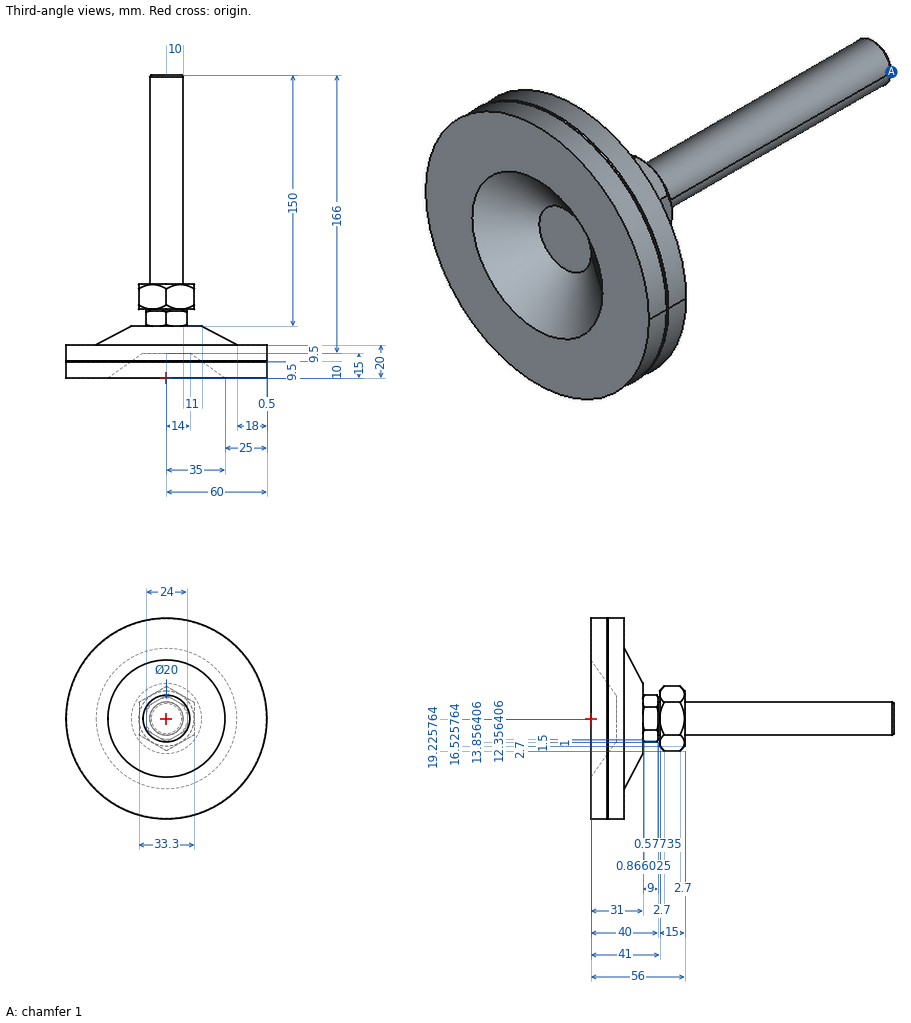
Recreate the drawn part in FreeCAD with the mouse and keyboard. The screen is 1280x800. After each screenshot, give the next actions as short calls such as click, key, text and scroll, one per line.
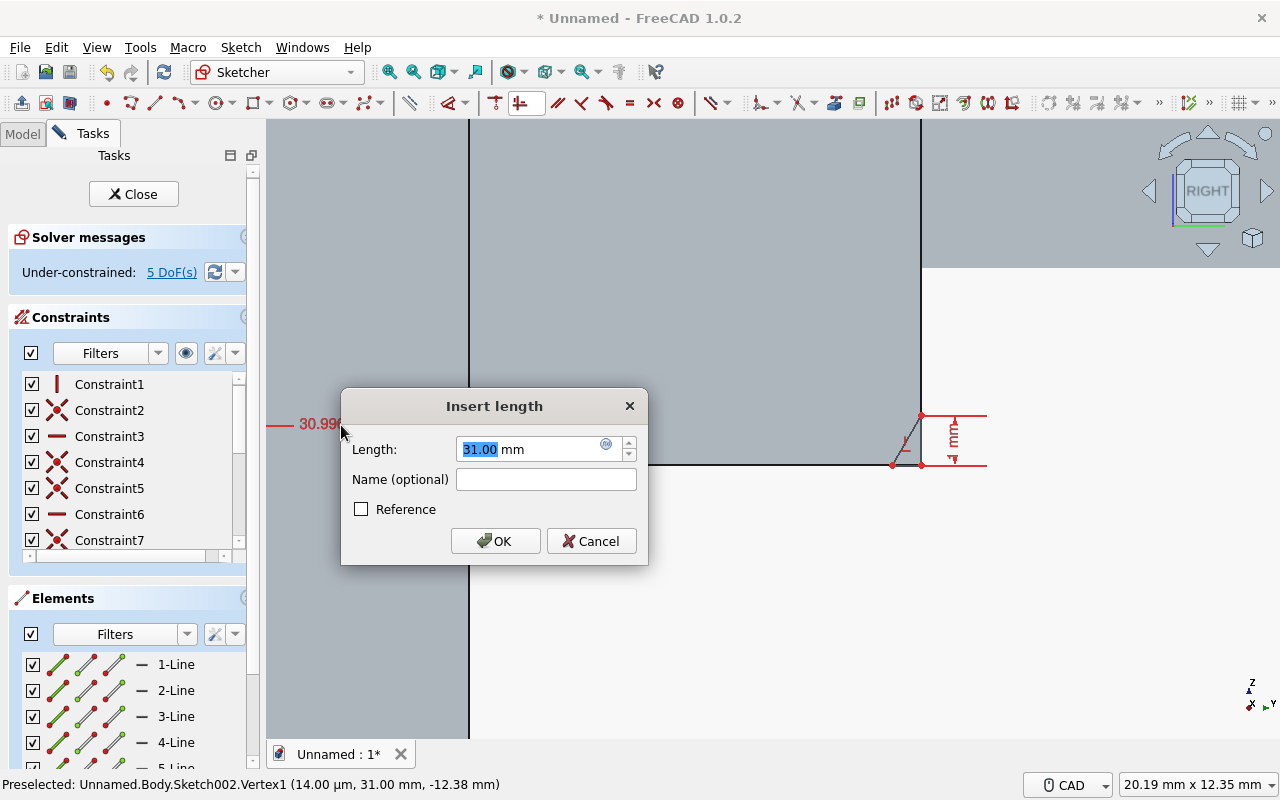
text(31)
key(Return)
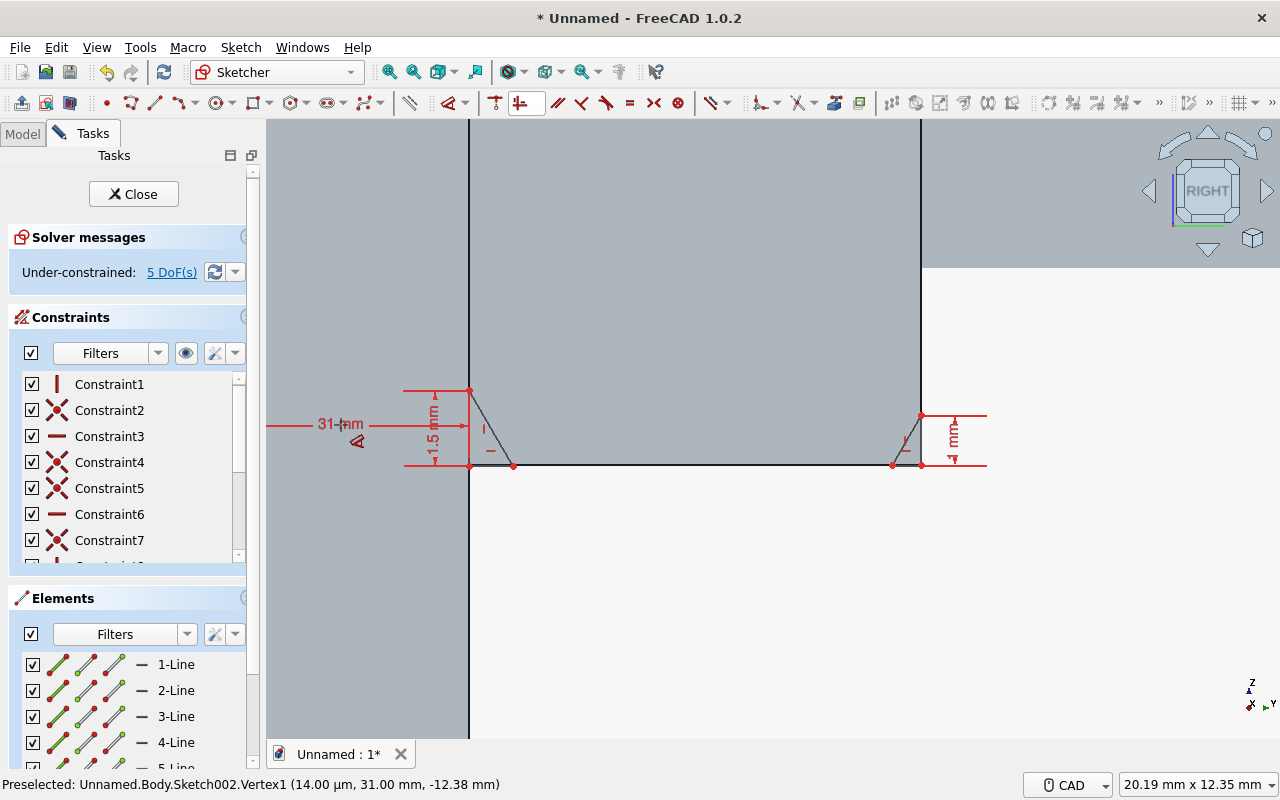
click(921, 466)
click(608, 500)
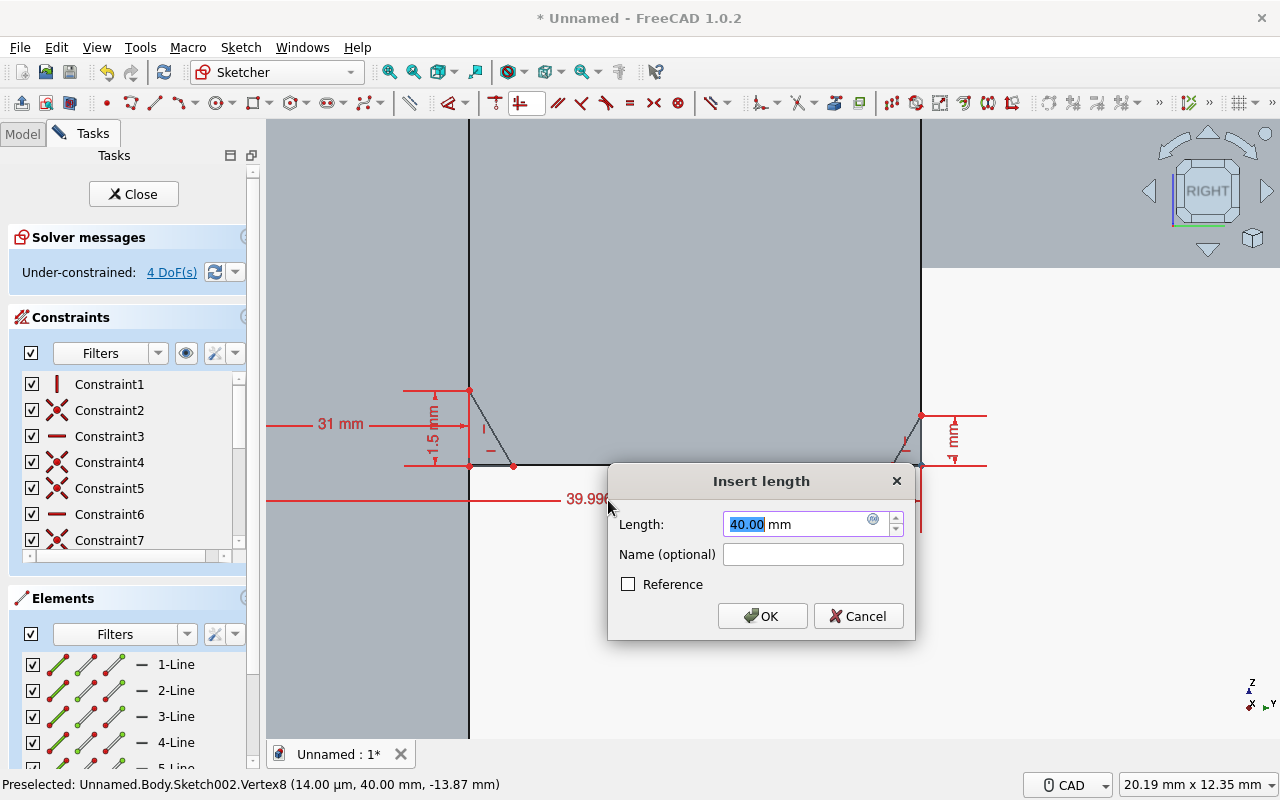
text(40)
key(Return)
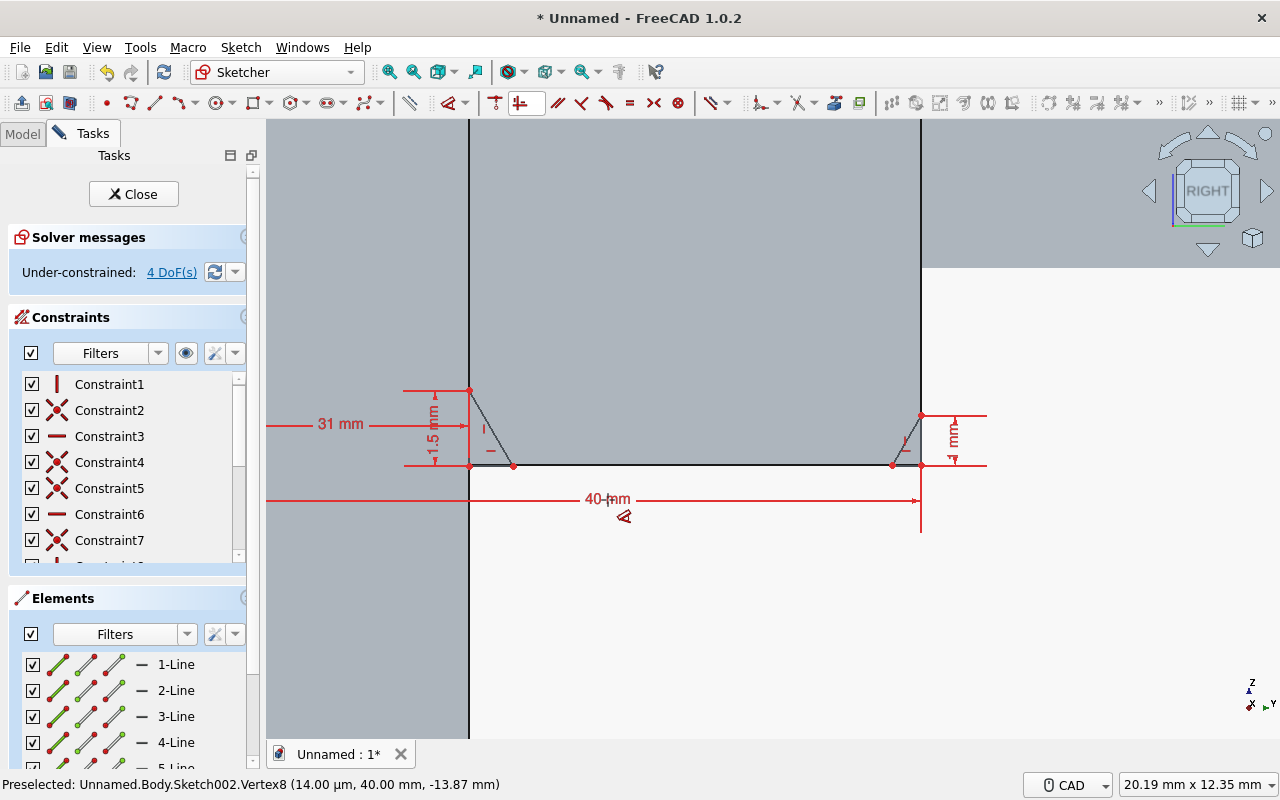
scroll(904, 466, up, 2)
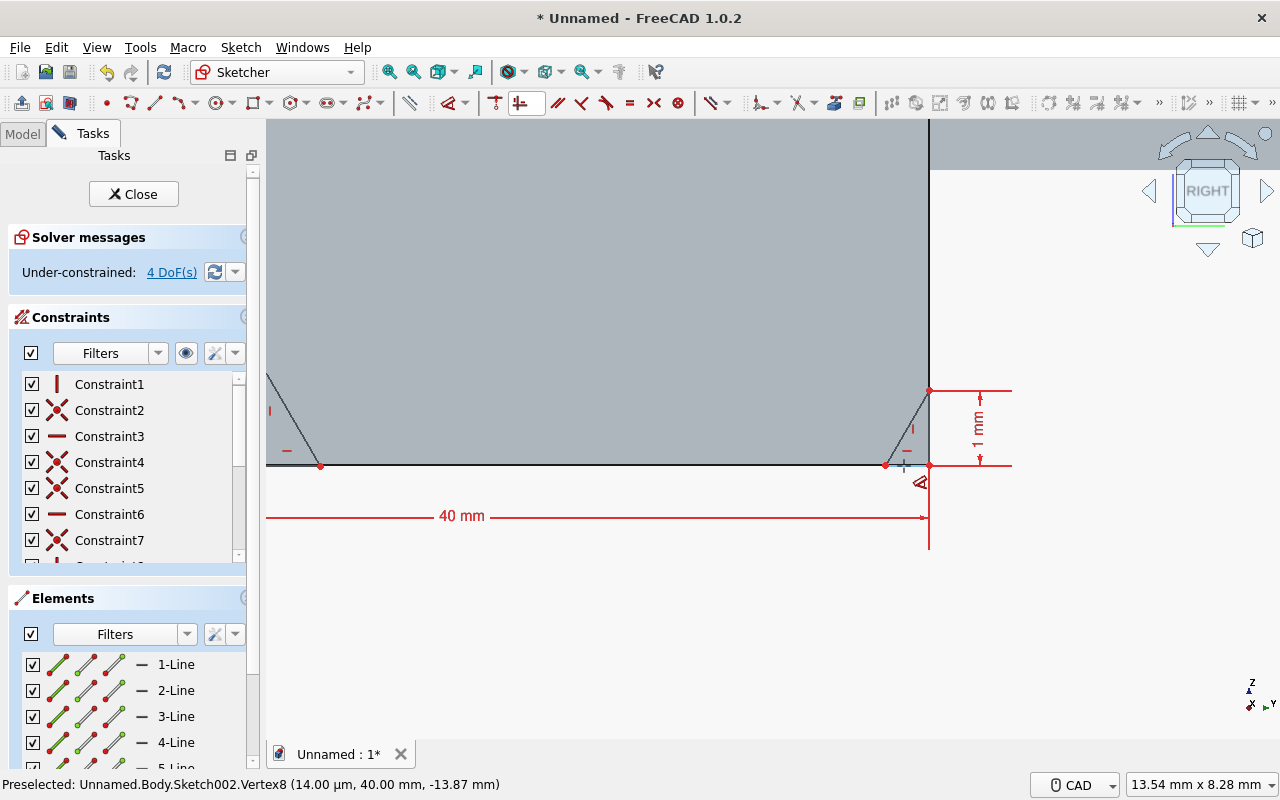
click(903, 466)
click(908, 500)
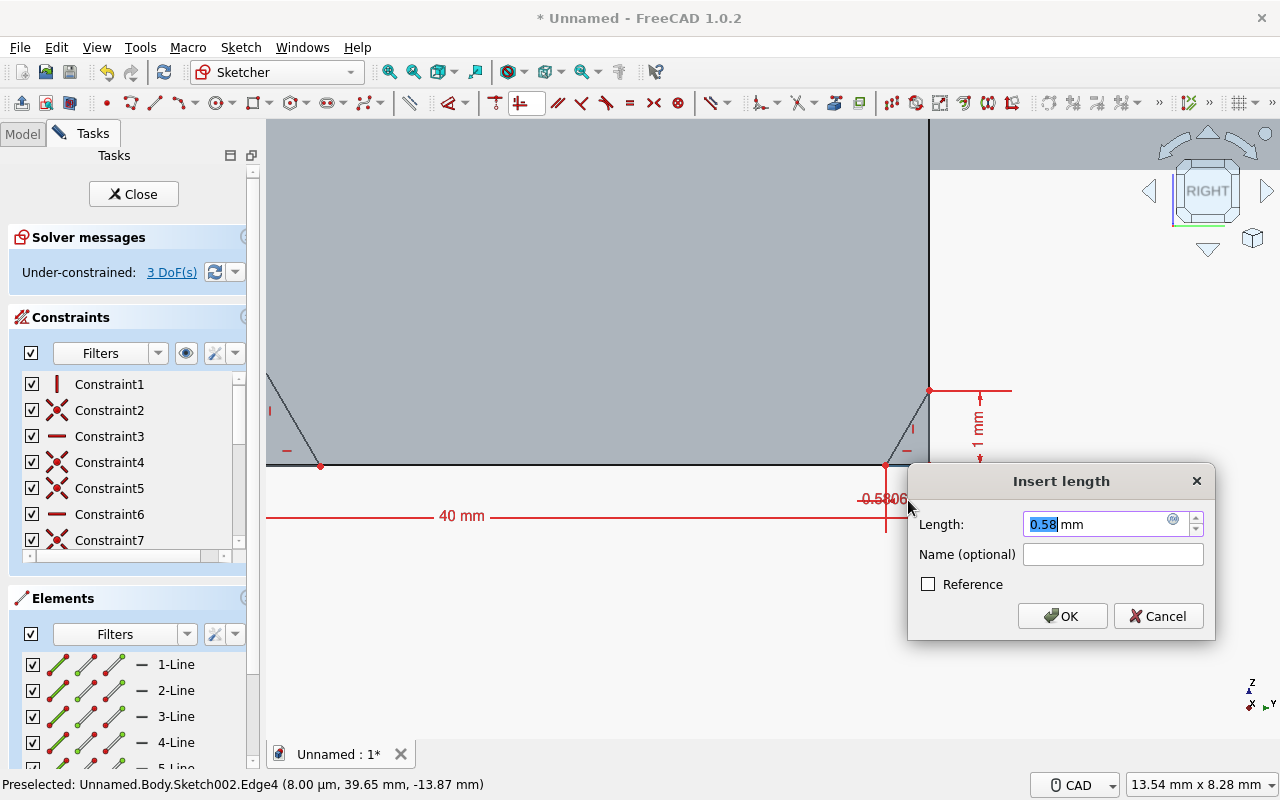
text(0.57735)
key(Return)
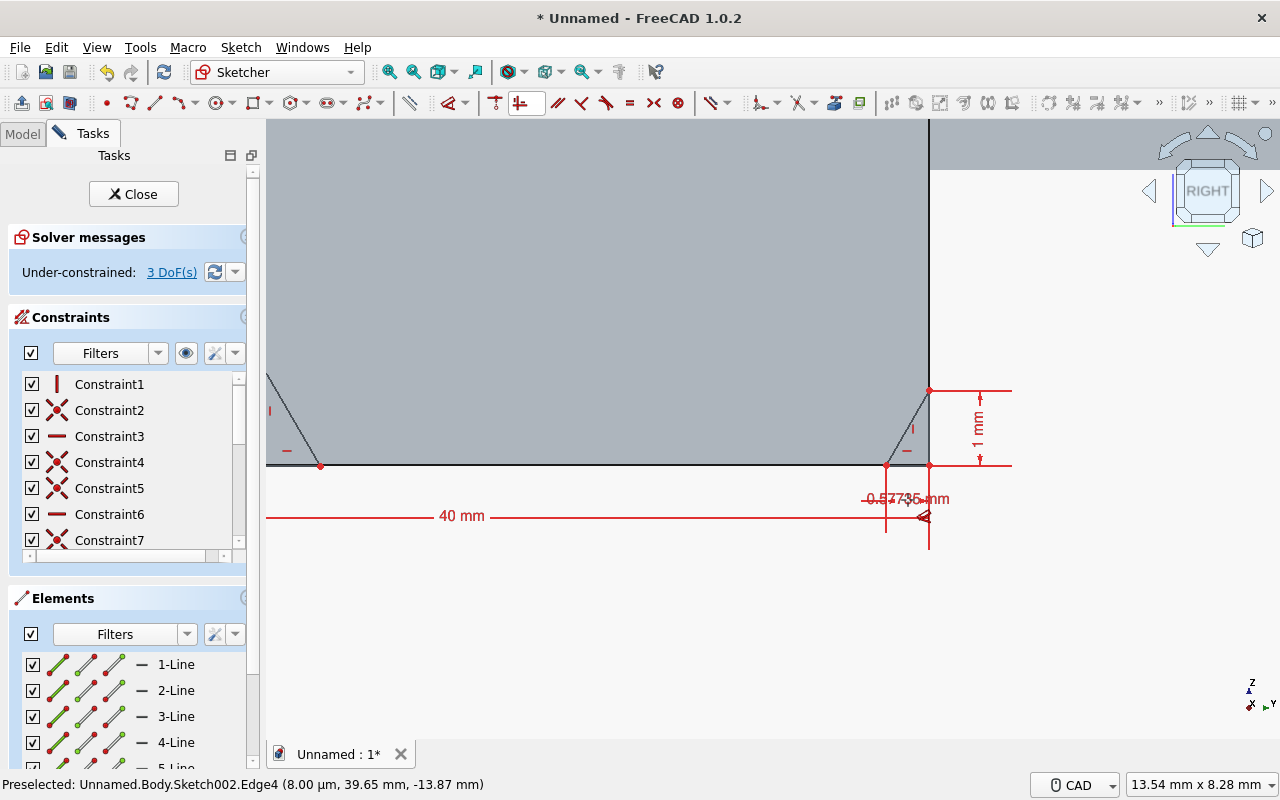
click(301, 466)
click(307, 500)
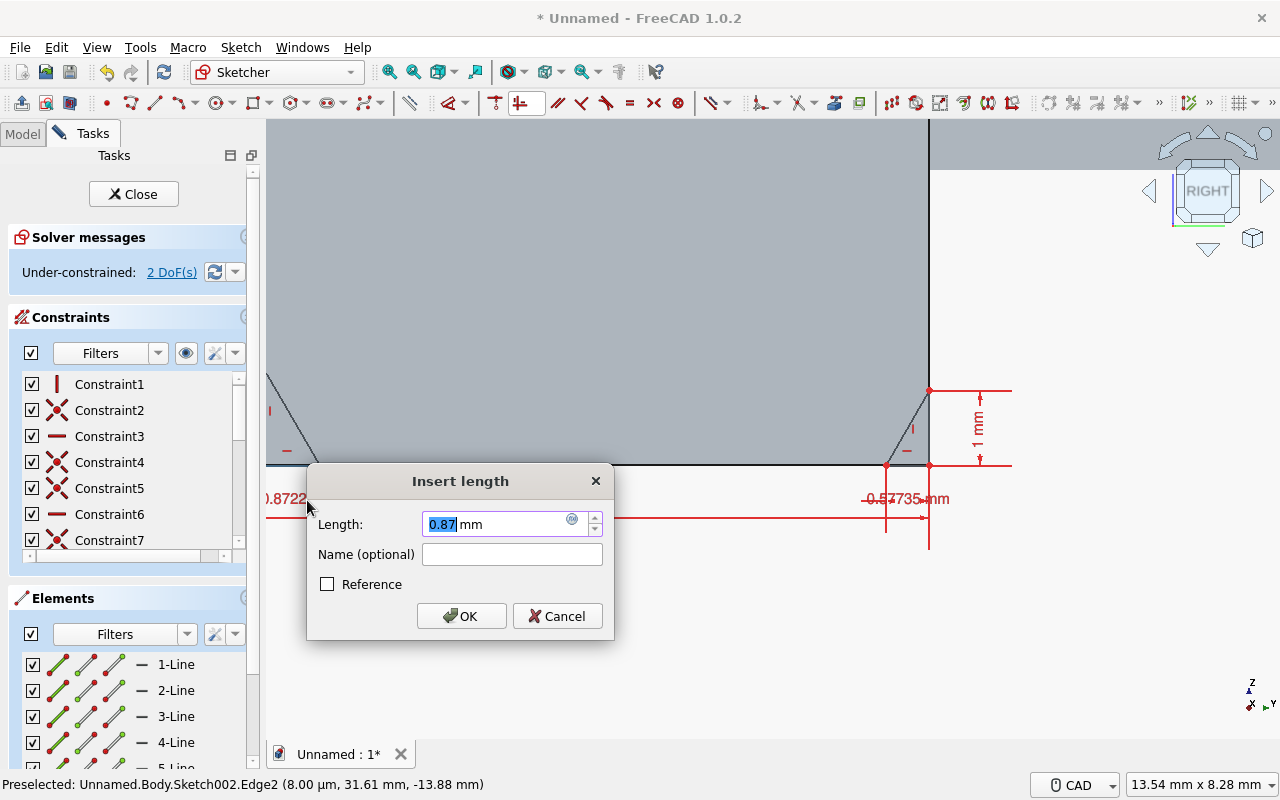
text(0.866025)
key(Return)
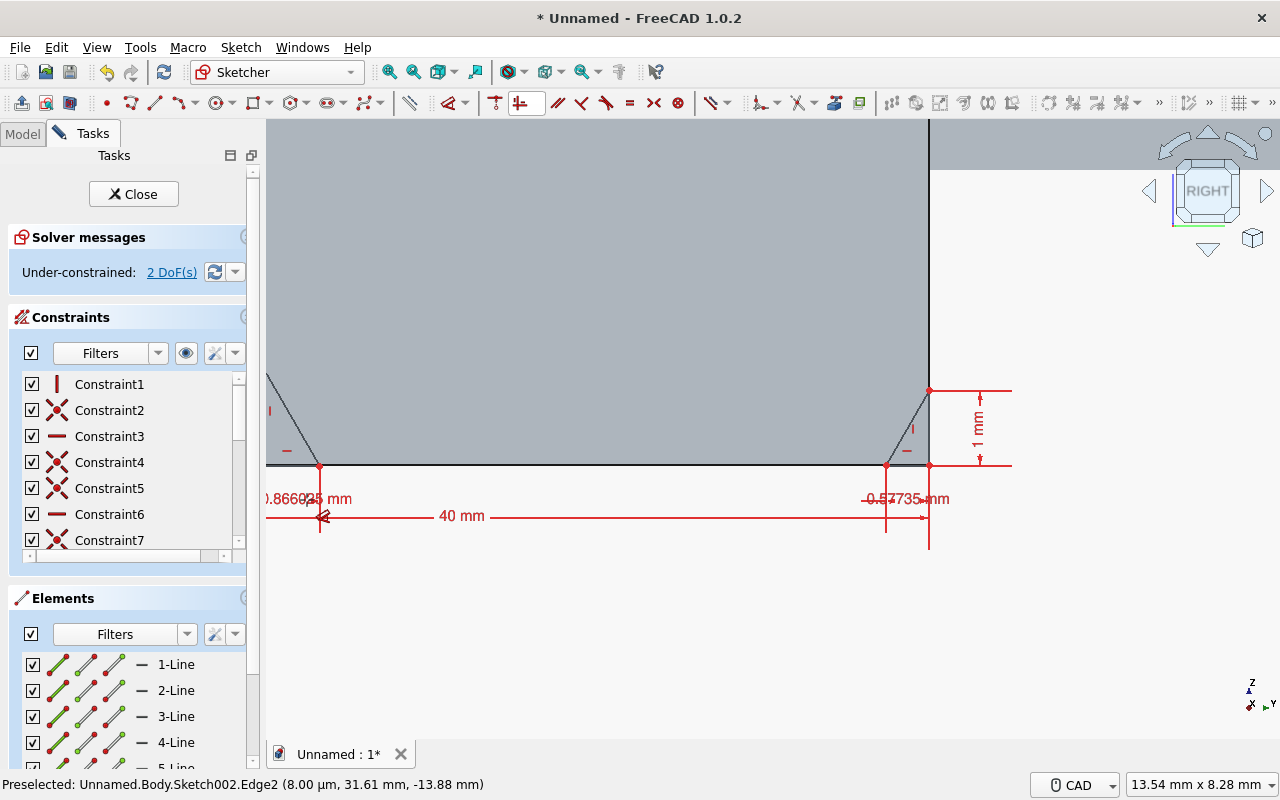
scroll(1115, 521, down, 1)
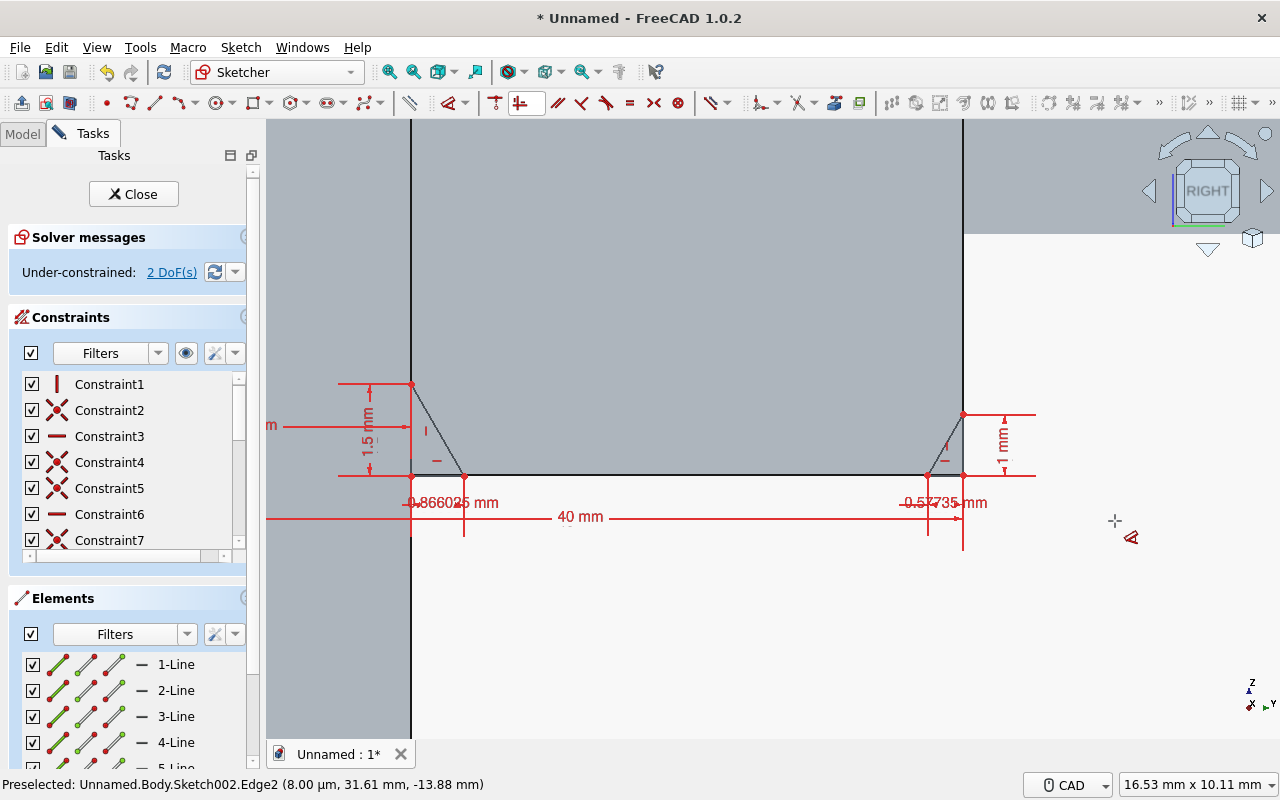
click(411, 384)
click(445, 266)